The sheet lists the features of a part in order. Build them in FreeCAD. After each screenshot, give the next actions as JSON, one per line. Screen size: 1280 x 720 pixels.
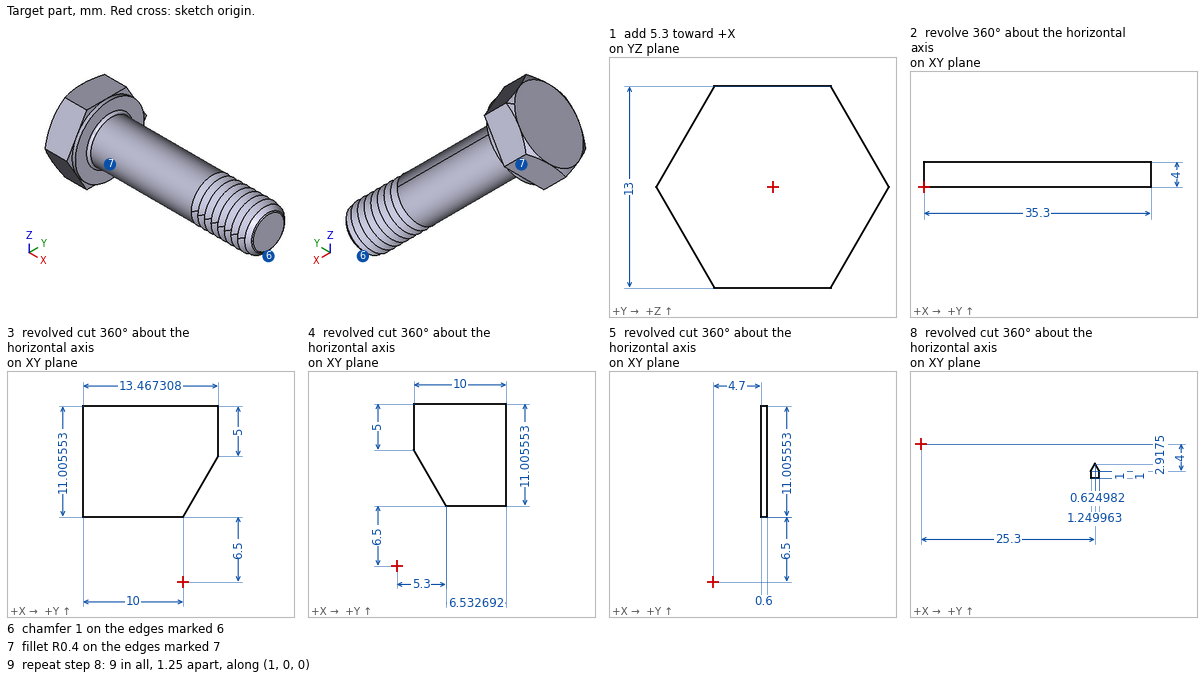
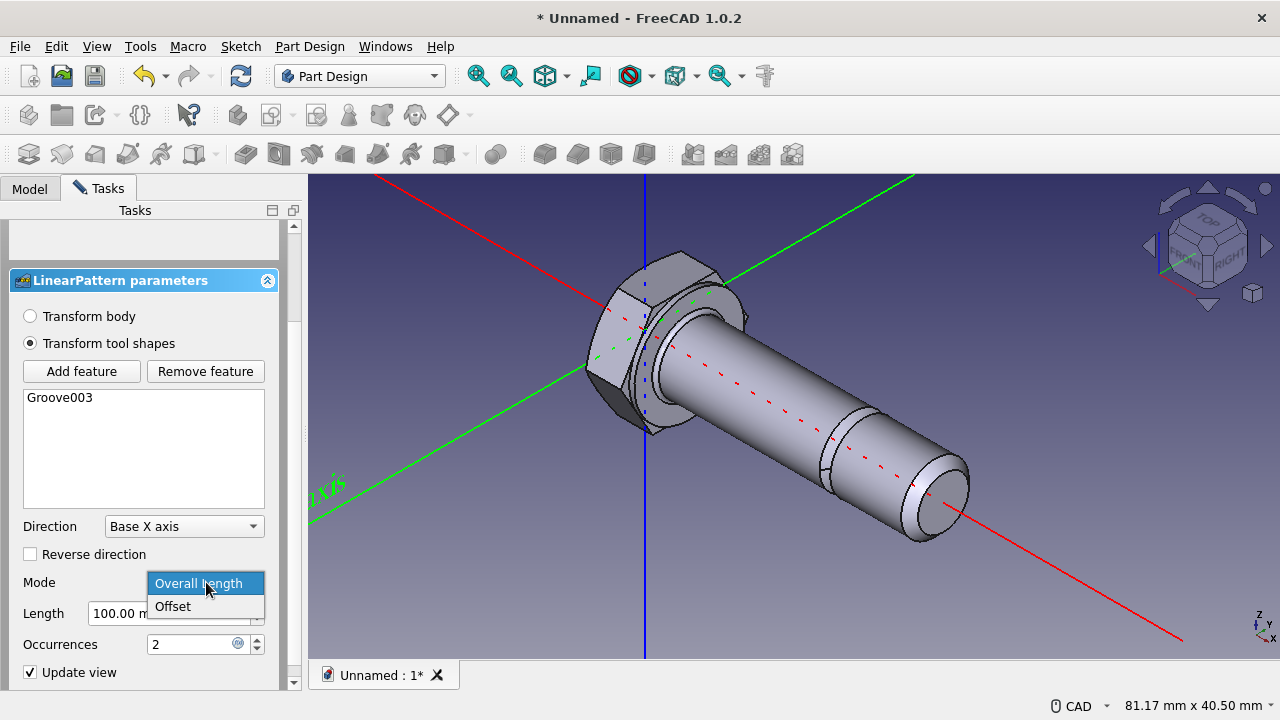
{"action": "left_click", "coordinate": [204, 606]}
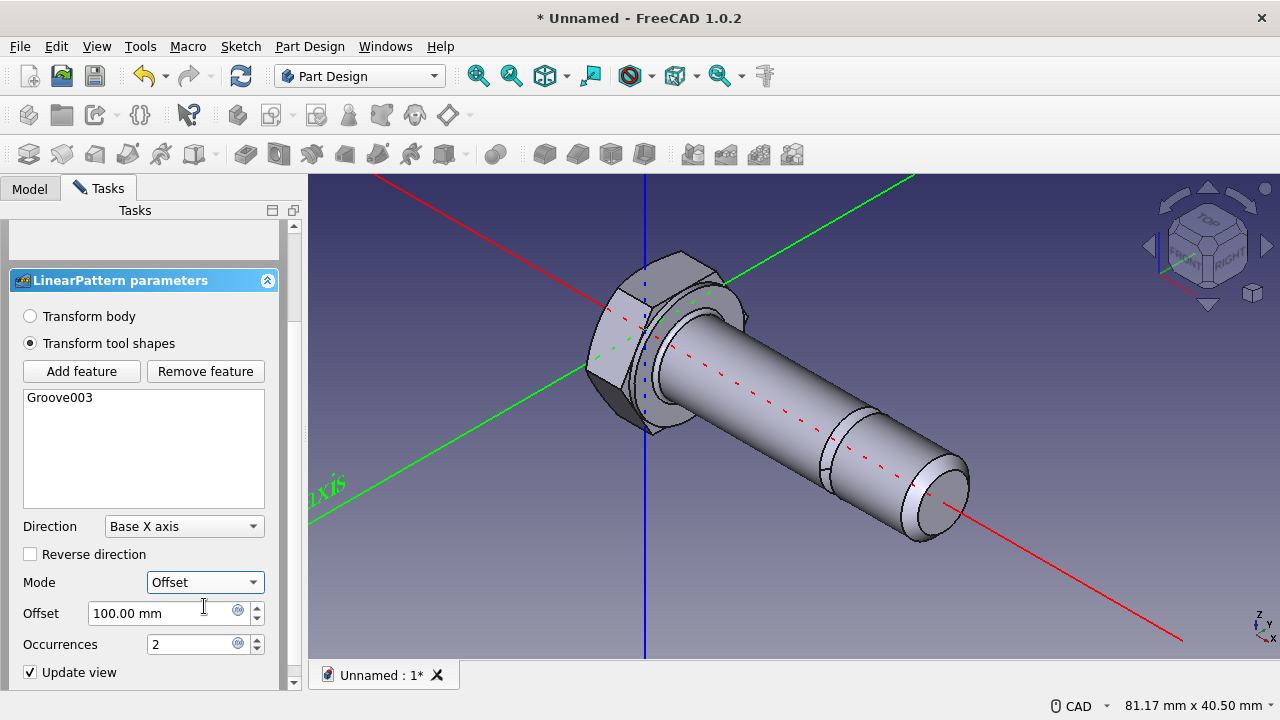
{"action": "triple_click", "coordinate": [170, 614]}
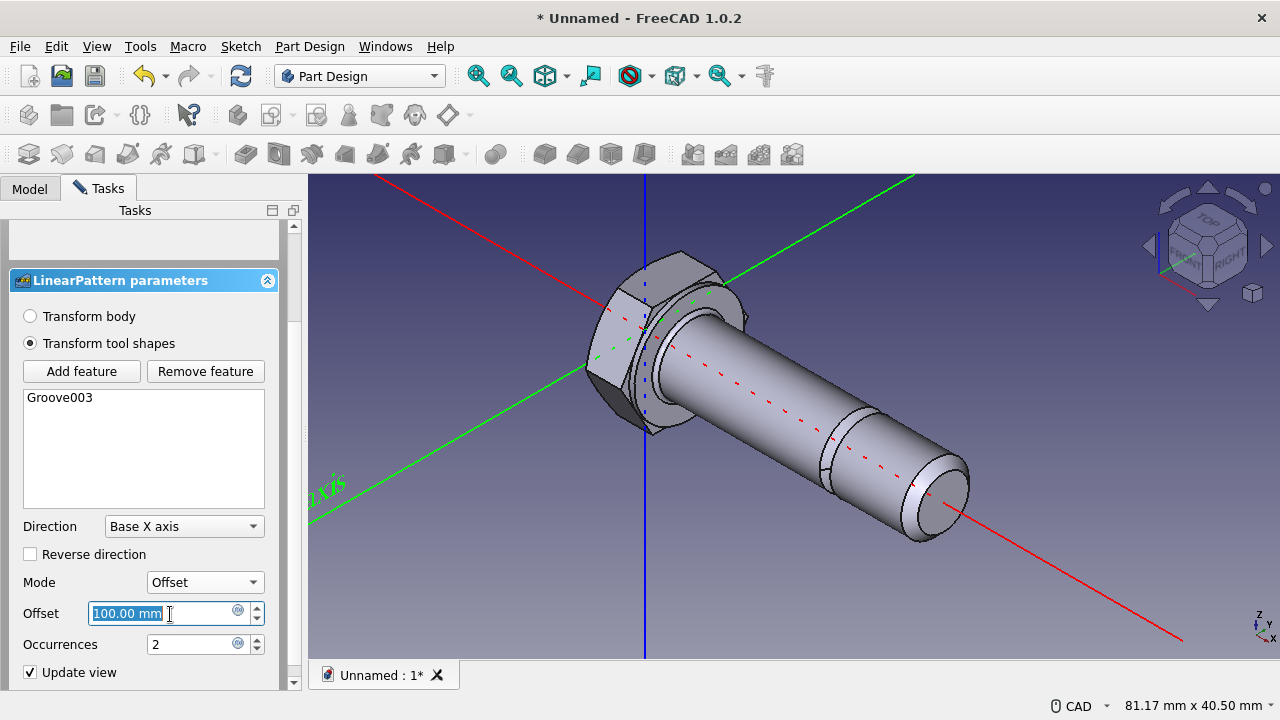
{"action": "type", "text": "1.25"}
{"action": "key", "text": "Tab"}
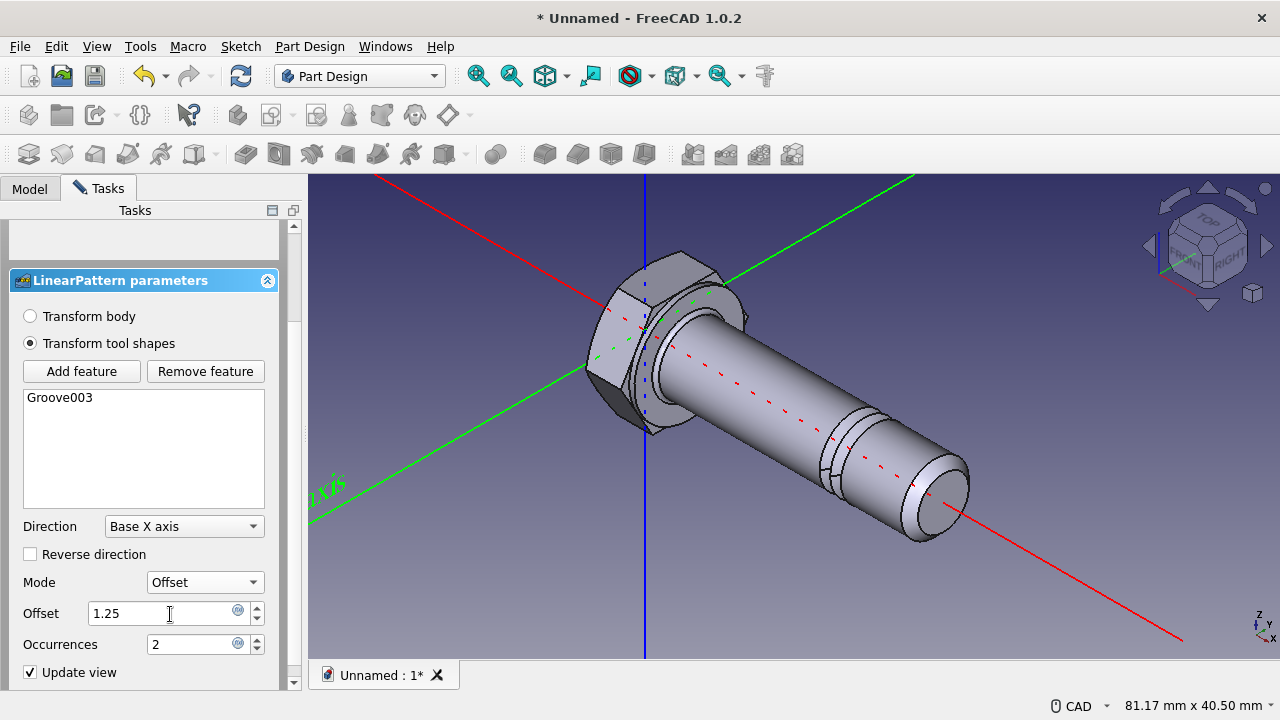
{"action": "triple_click", "coordinate": [199, 644]}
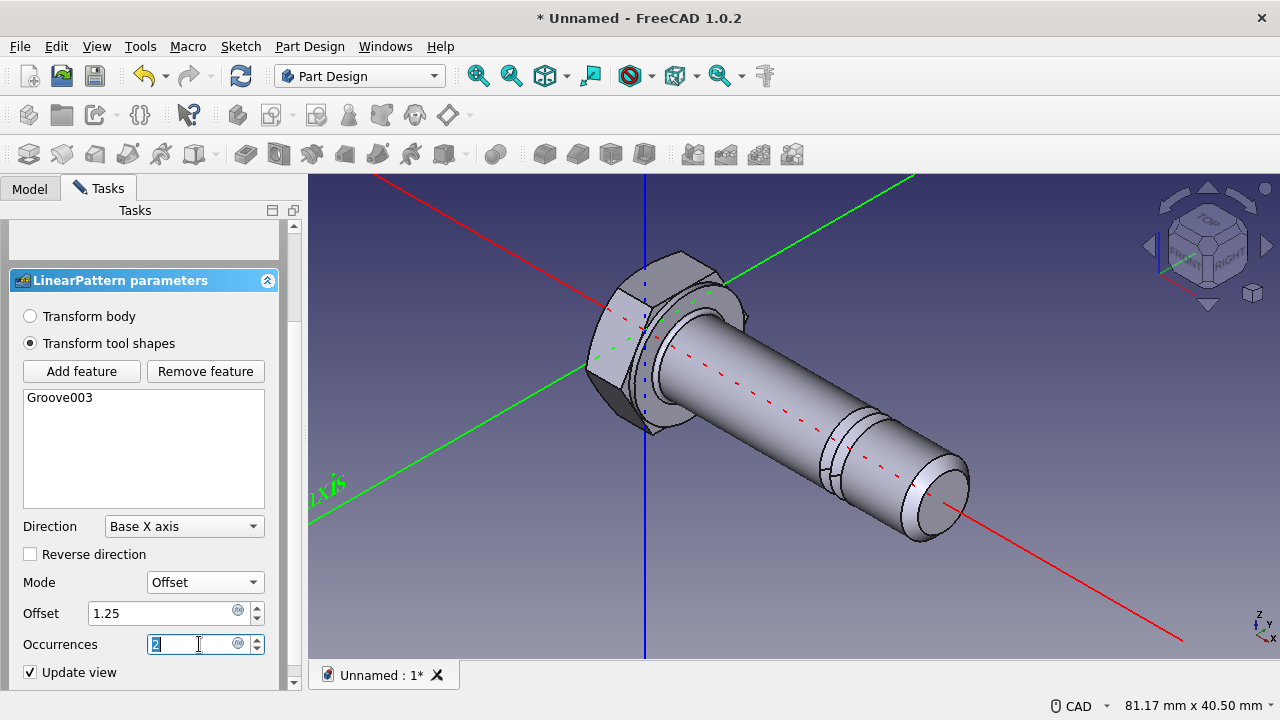
{"action": "type", "text": "9"}
{"action": "key", "text": "Tab"}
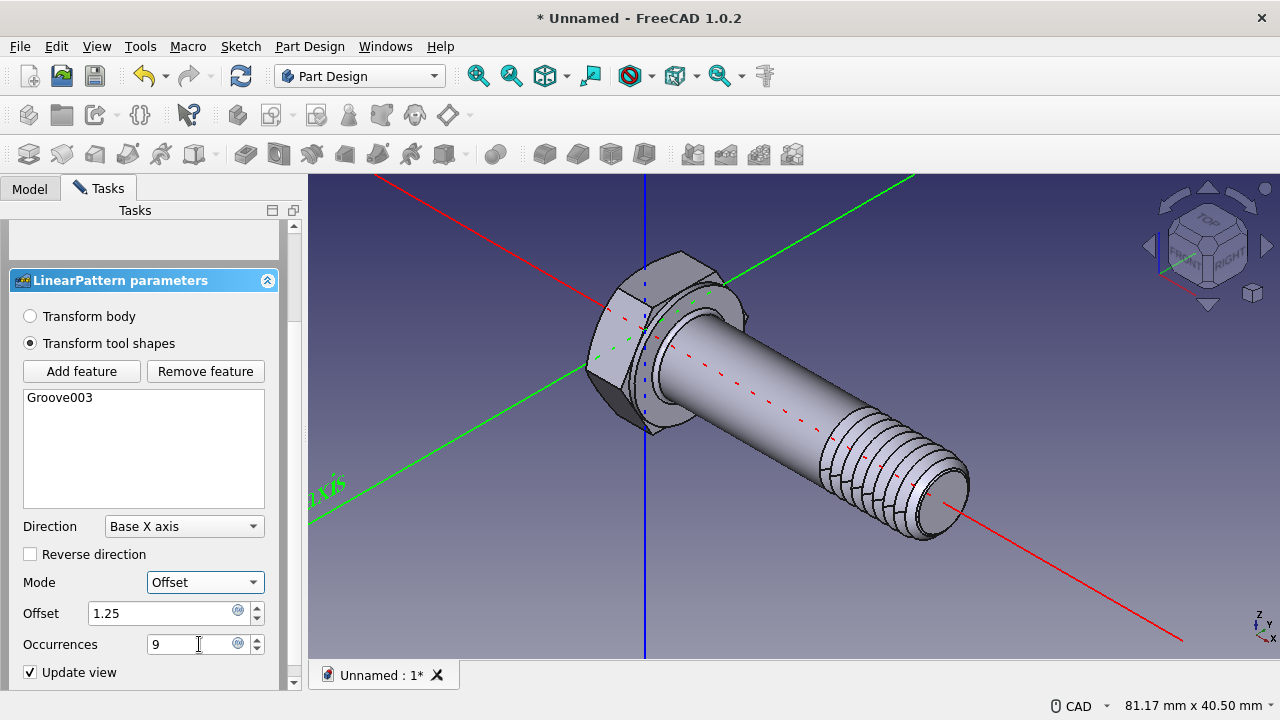
{"action": "scroll", "coordinate": [294, 455], "scroll_direction": "up", "scroll_amount": 3}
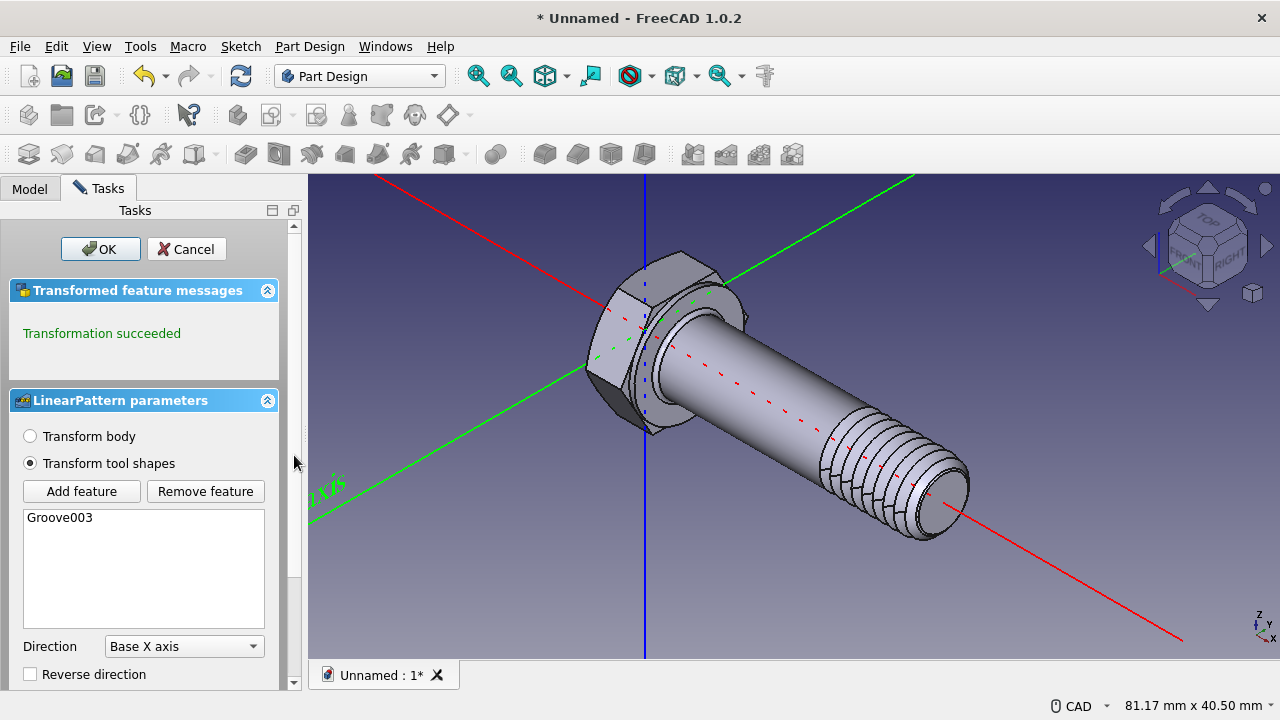
{"action": "left_click", "coordinate": [101, 249]}